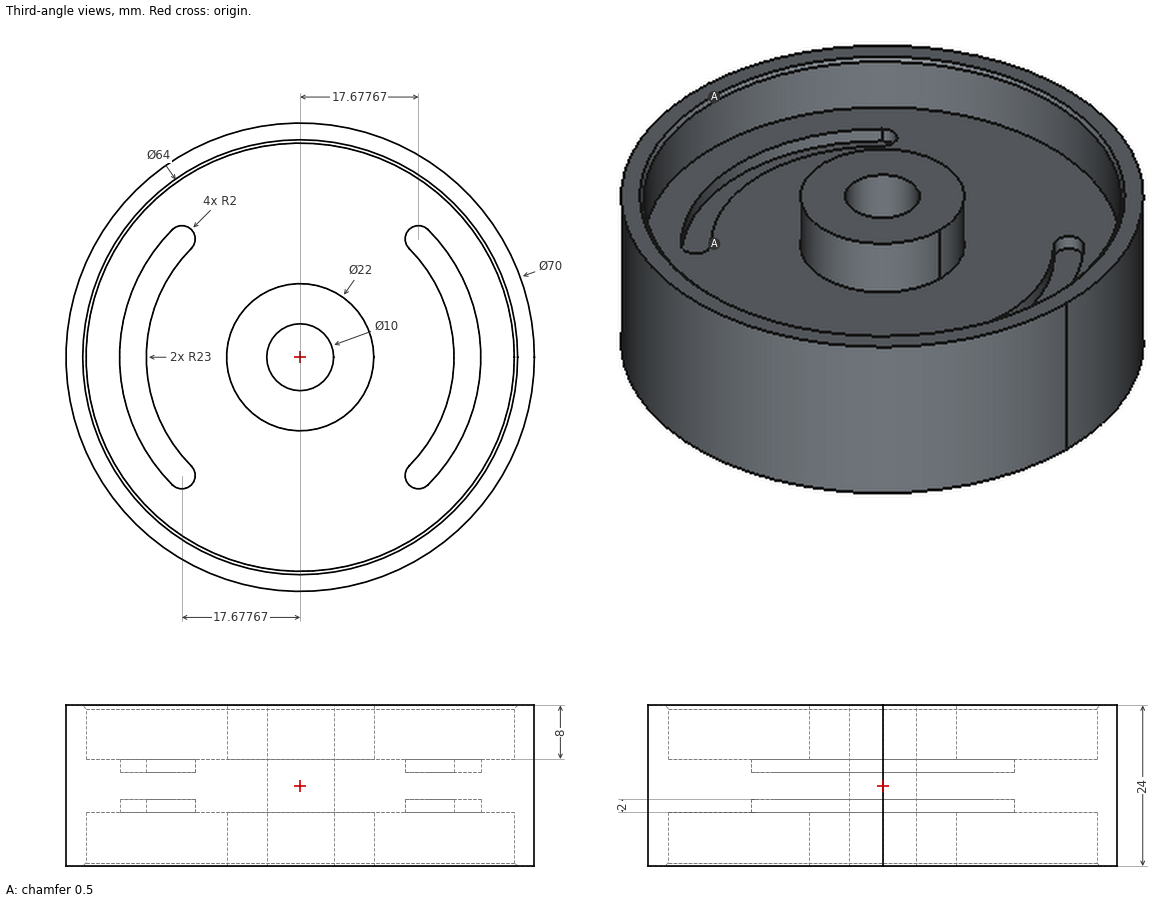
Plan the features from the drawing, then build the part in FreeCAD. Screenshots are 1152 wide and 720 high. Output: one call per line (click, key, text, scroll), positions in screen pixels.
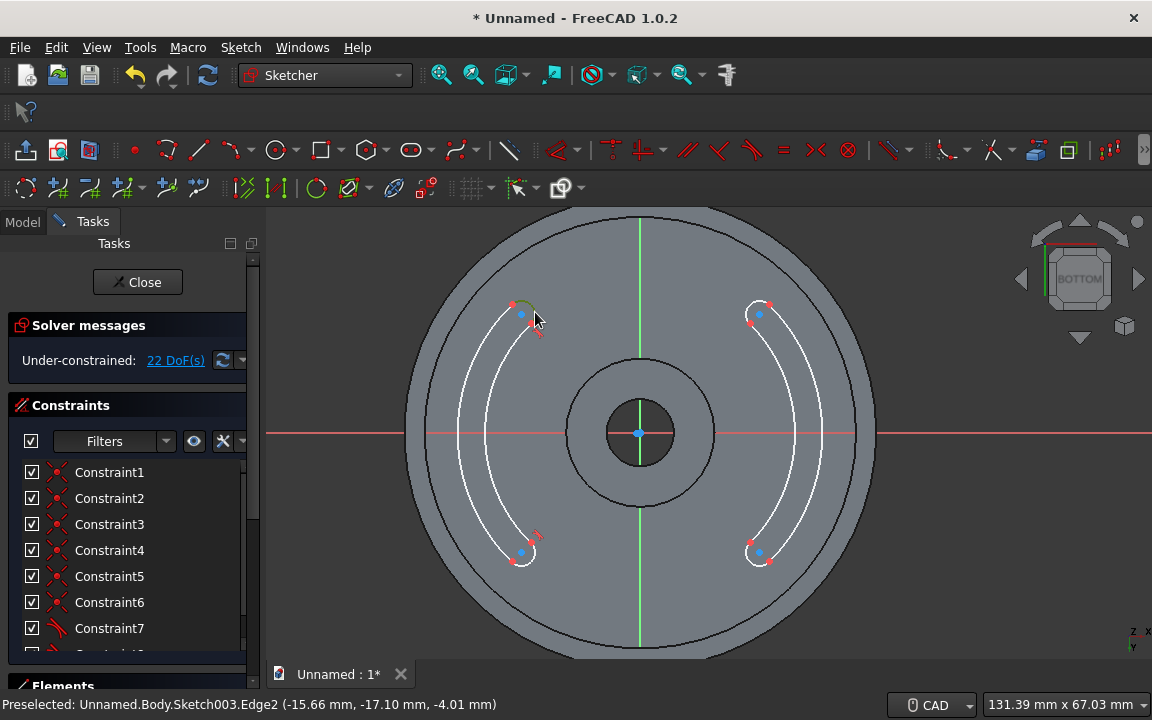
click(467, 377)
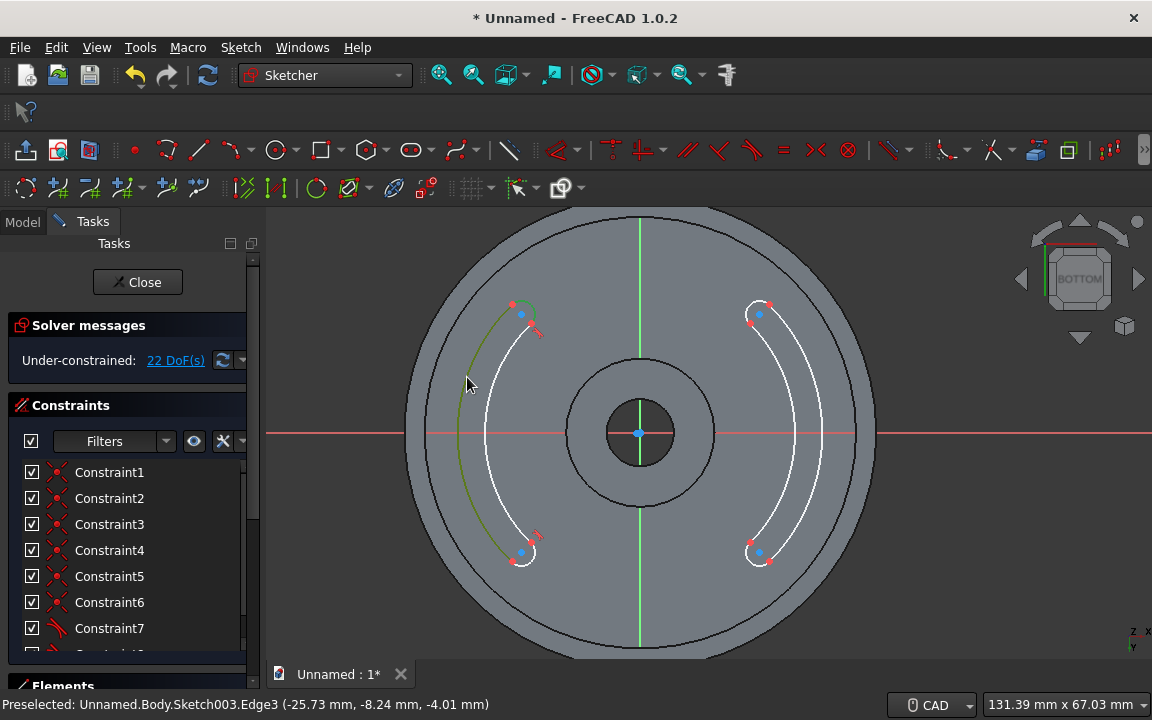
key(t)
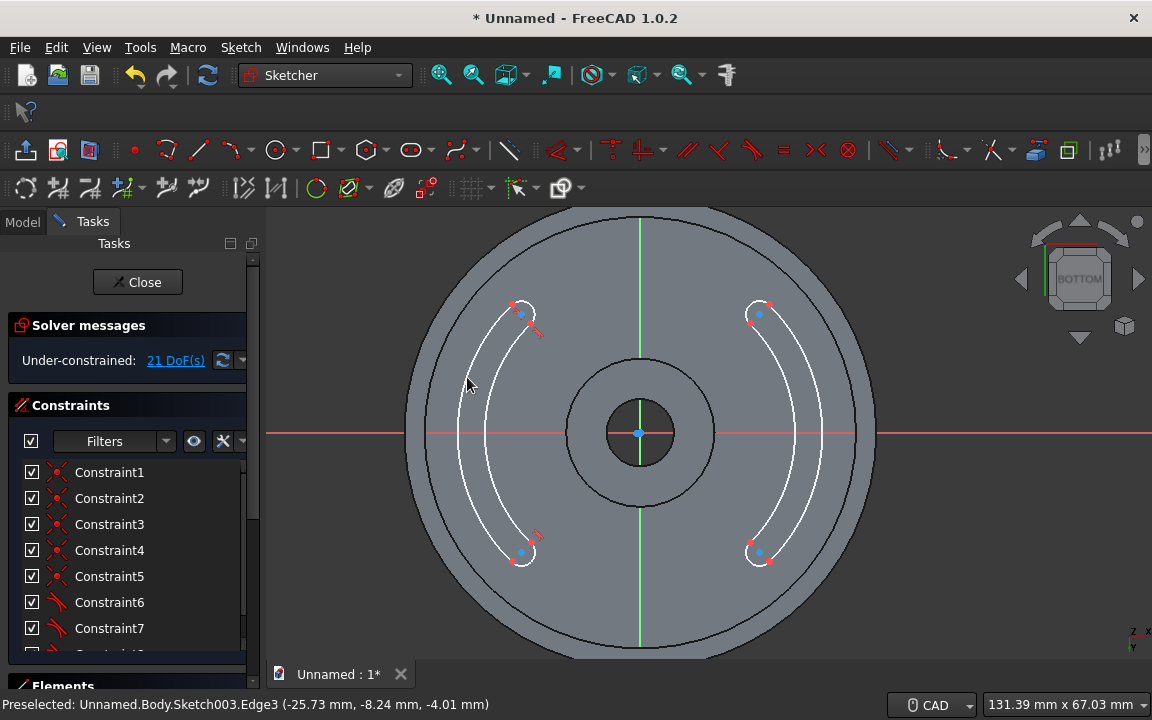
click(467, 377)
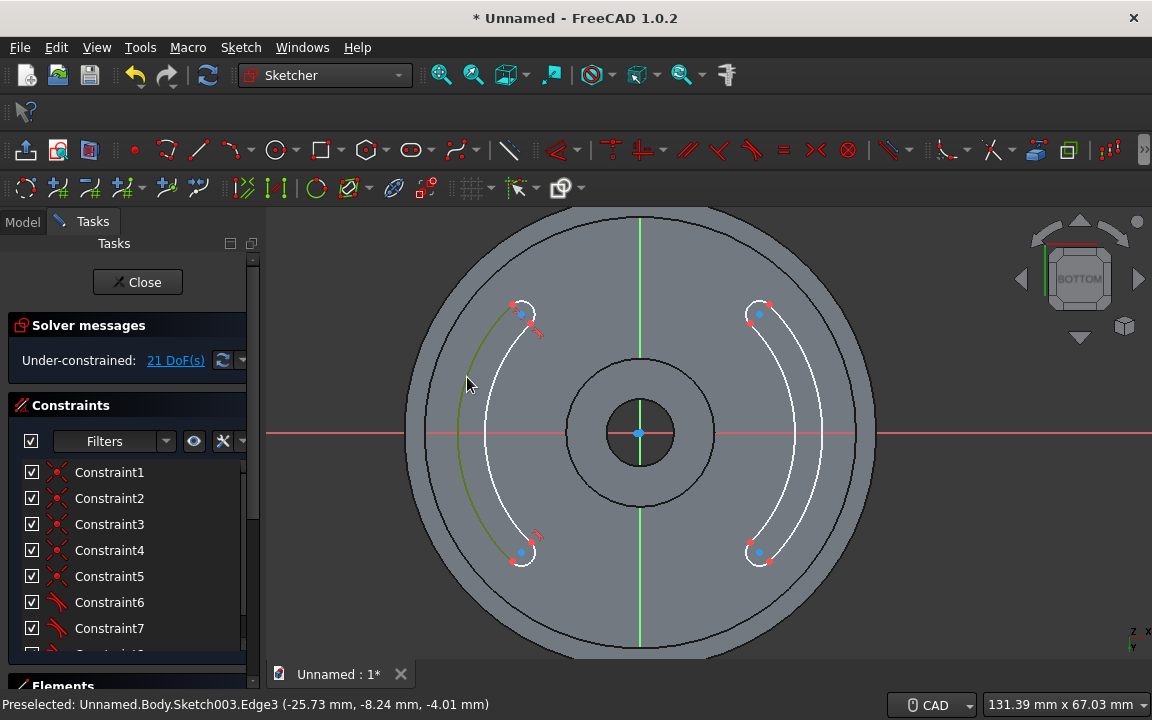
click(524, 566)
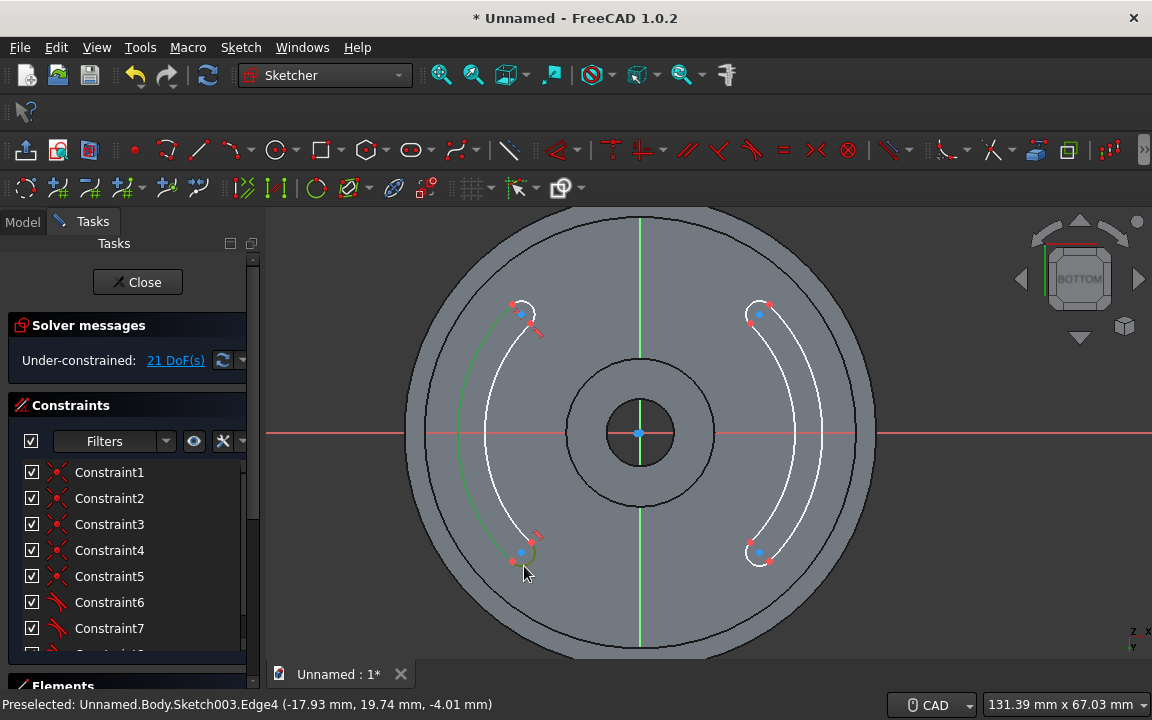
key(t)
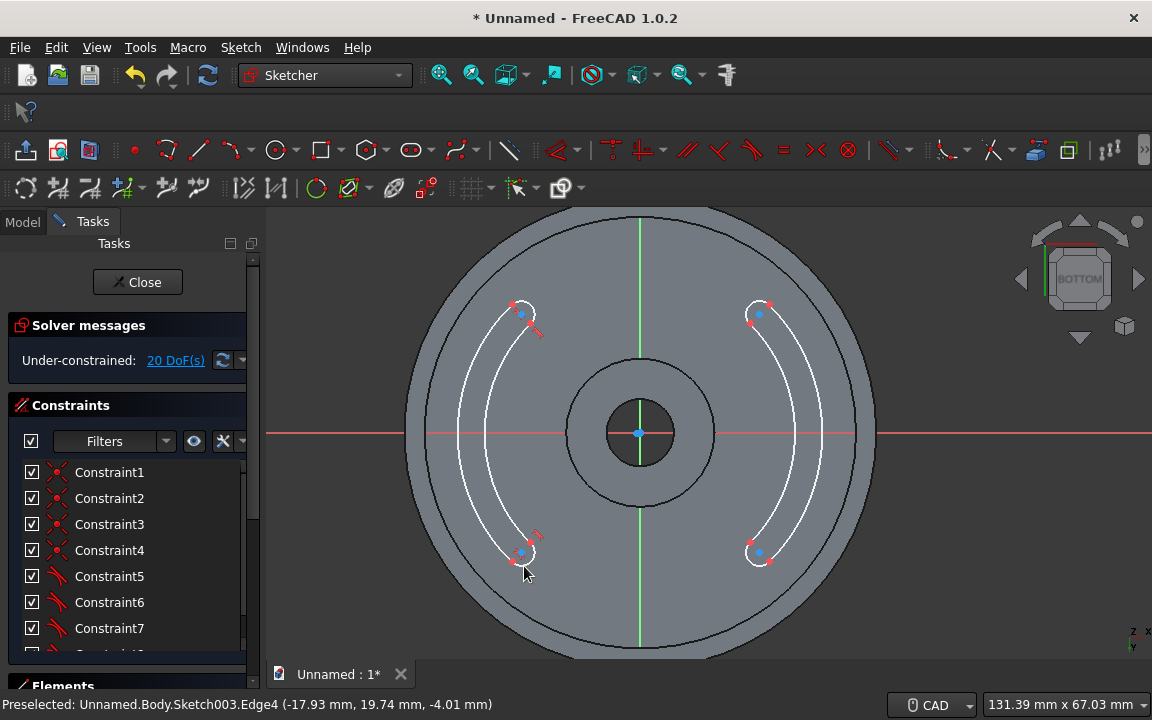
click(787, 481)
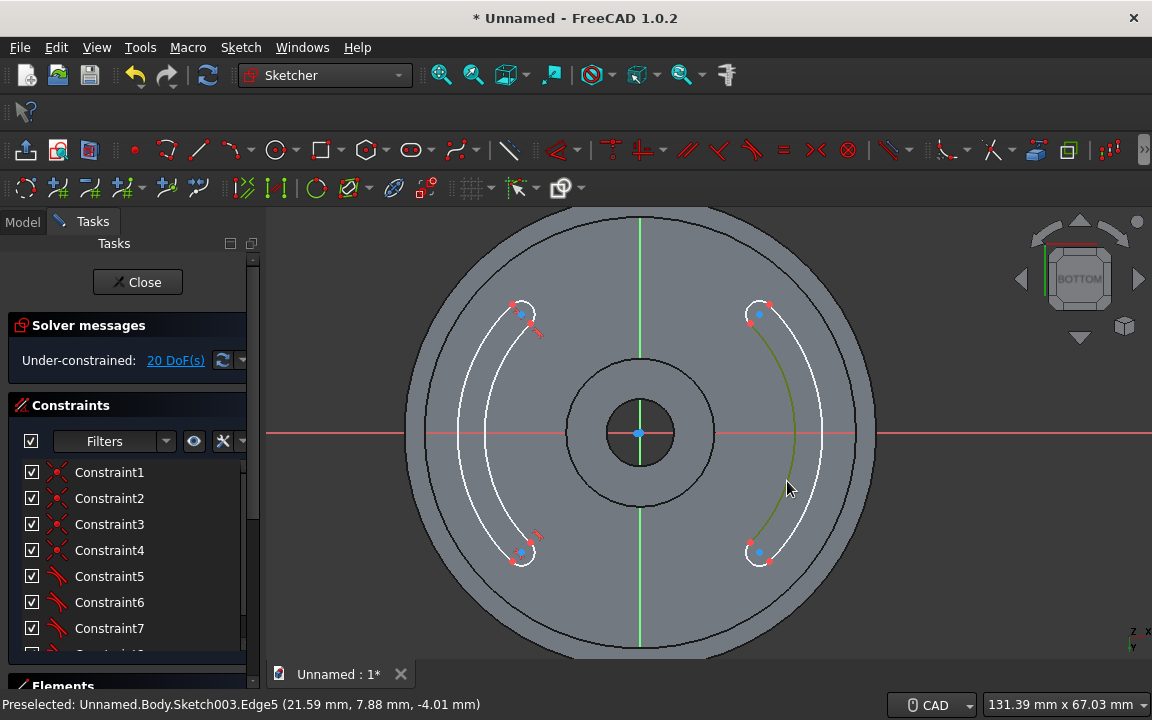
click(746, 555)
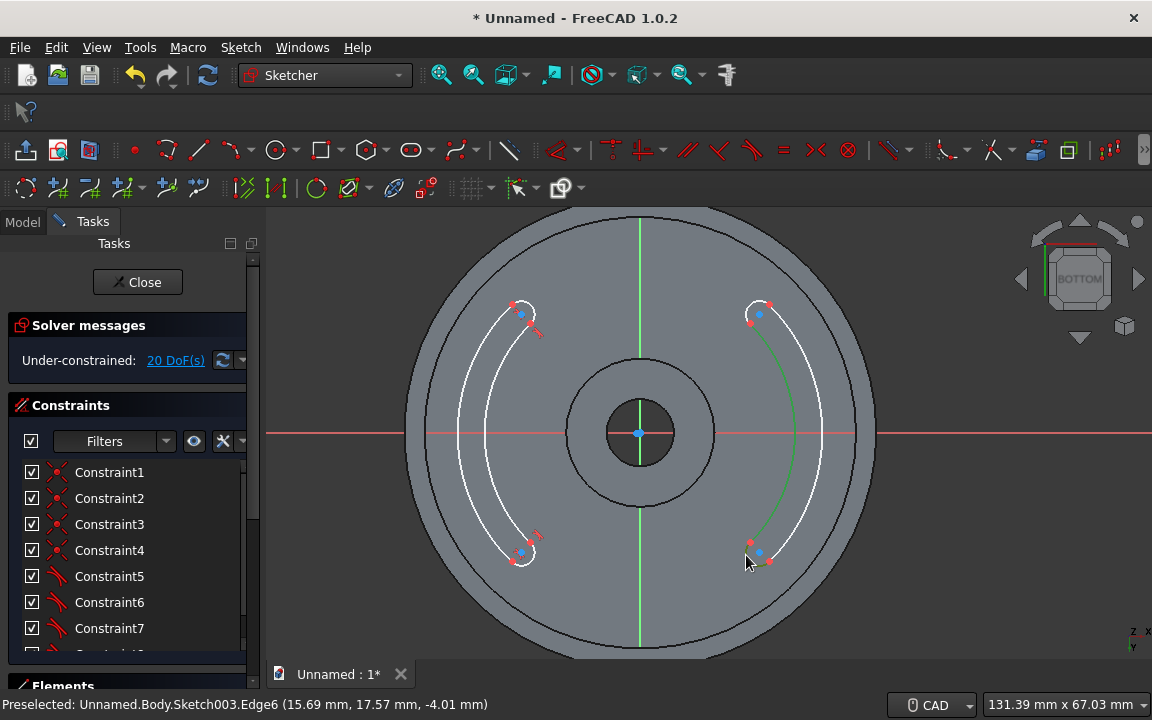
key(t)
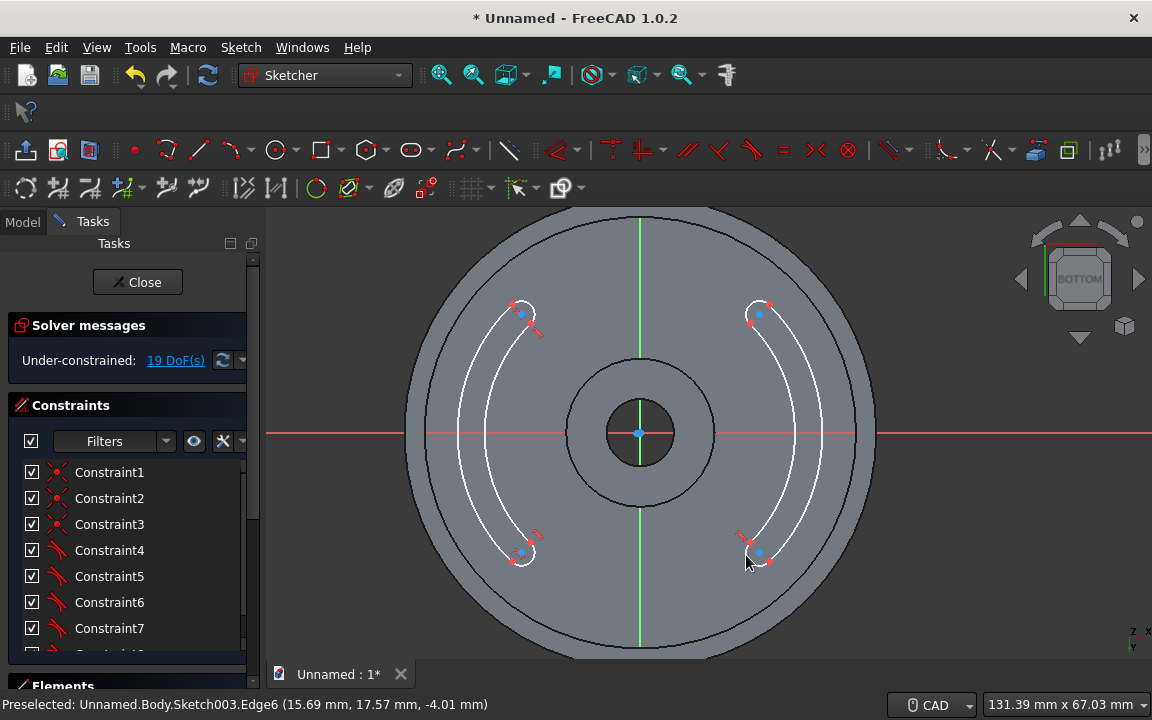
click(787, 481)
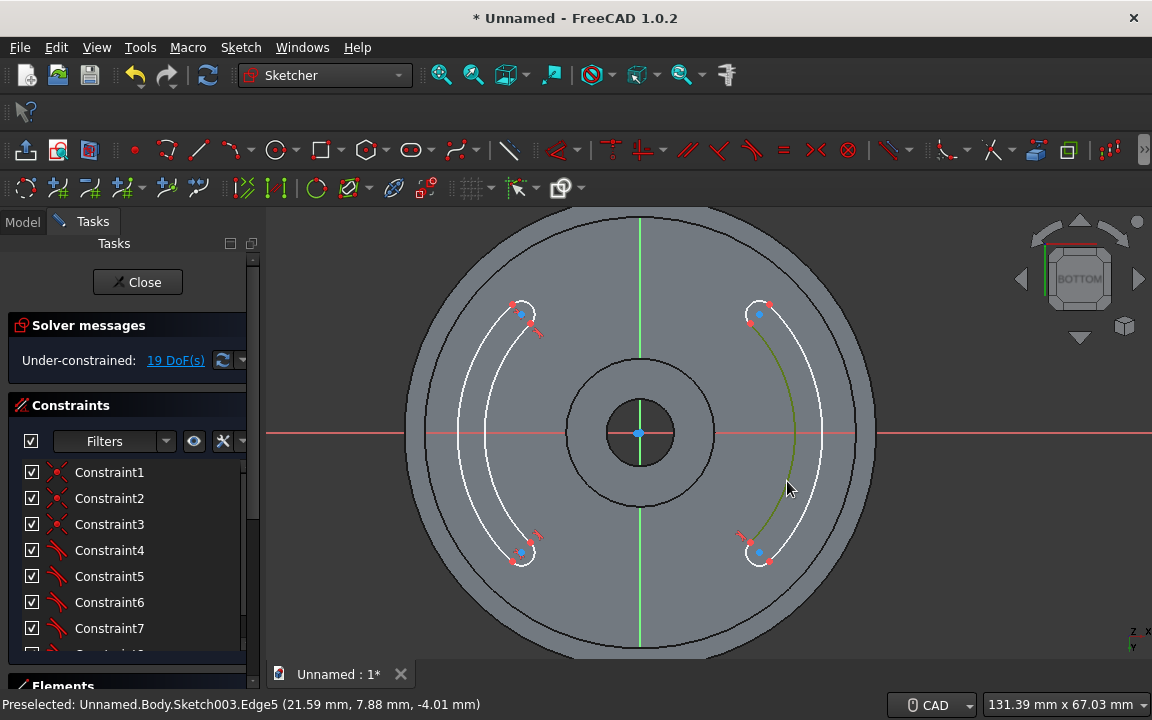
click(757, 301)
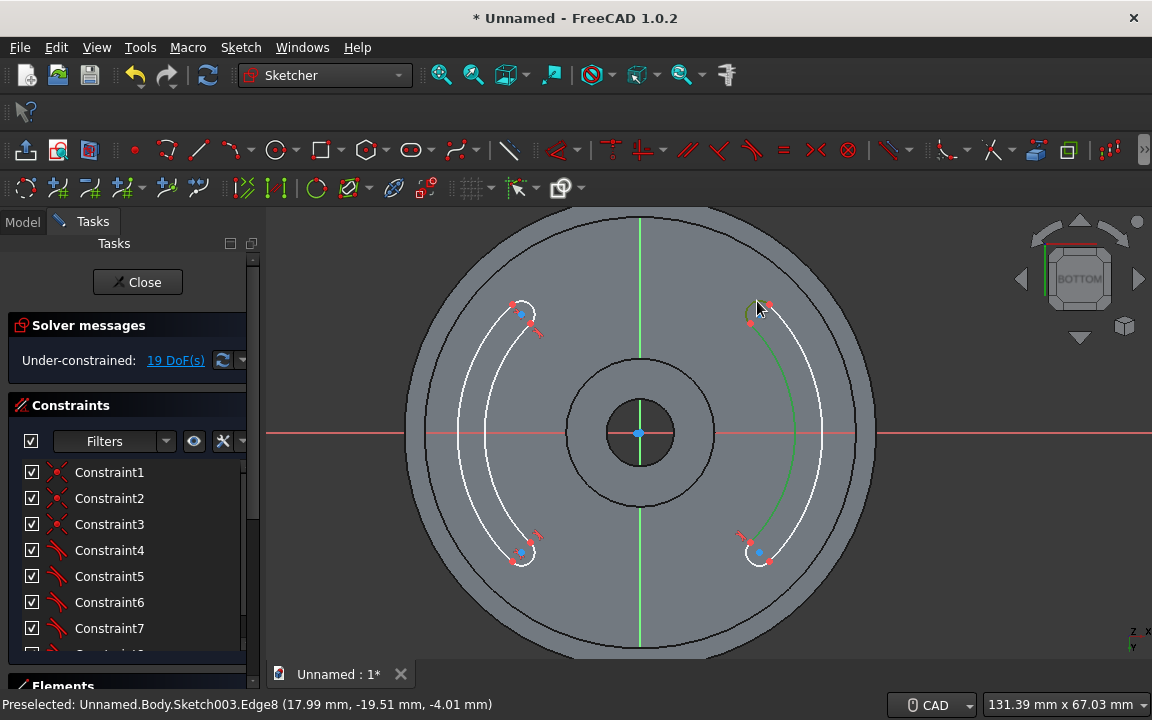
key(t)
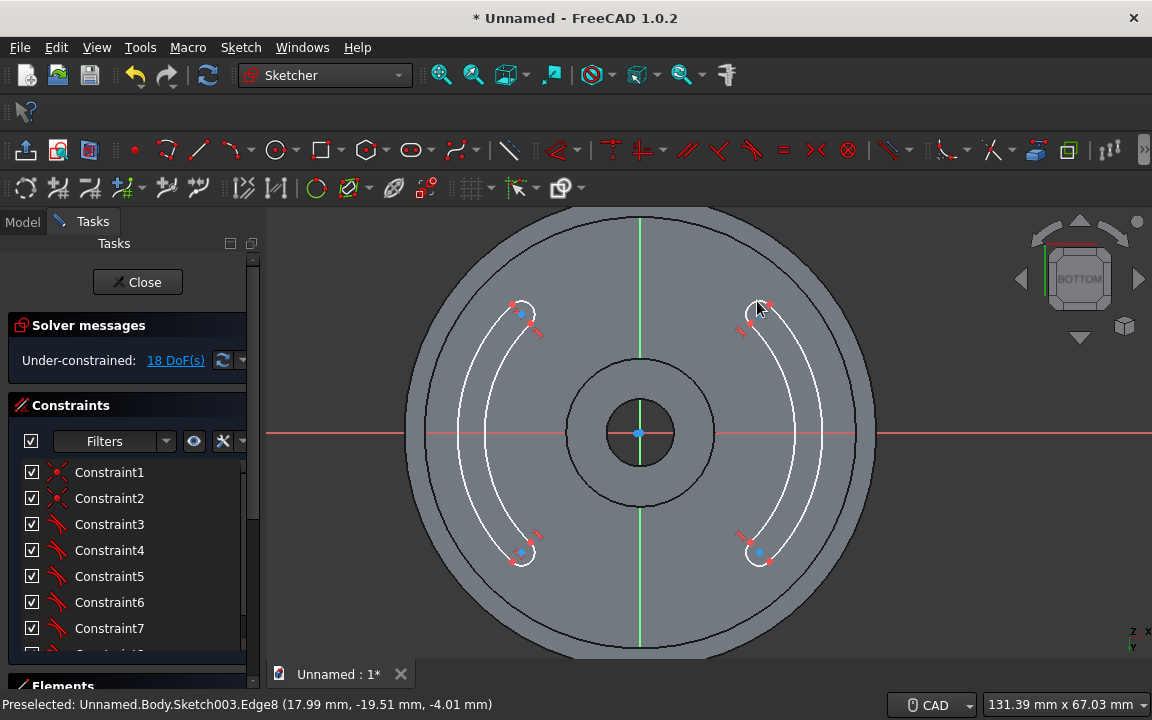
click(746, 555)